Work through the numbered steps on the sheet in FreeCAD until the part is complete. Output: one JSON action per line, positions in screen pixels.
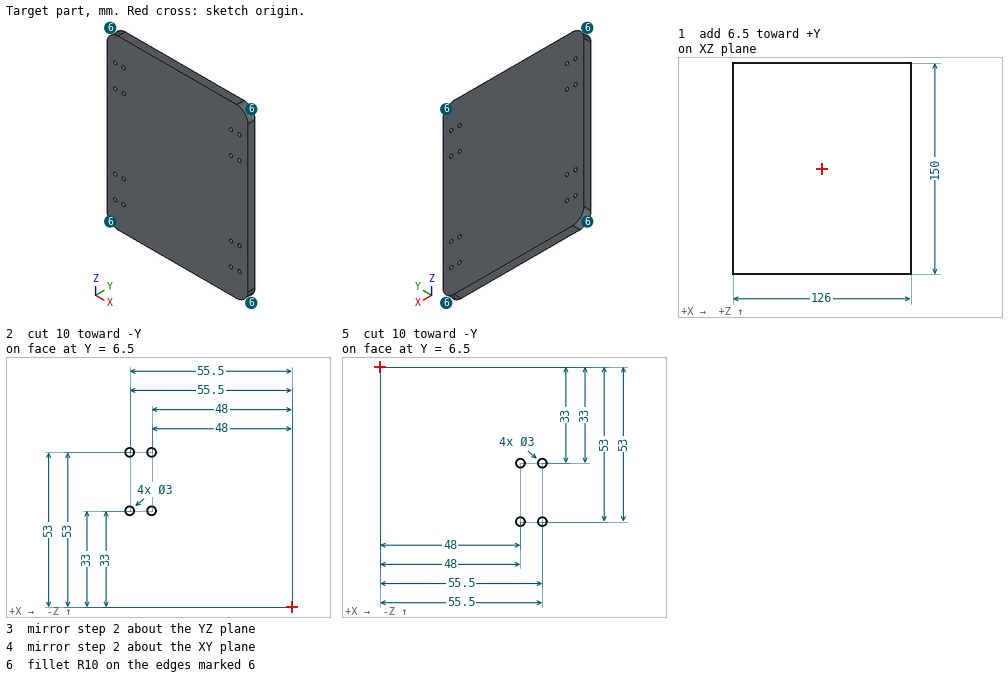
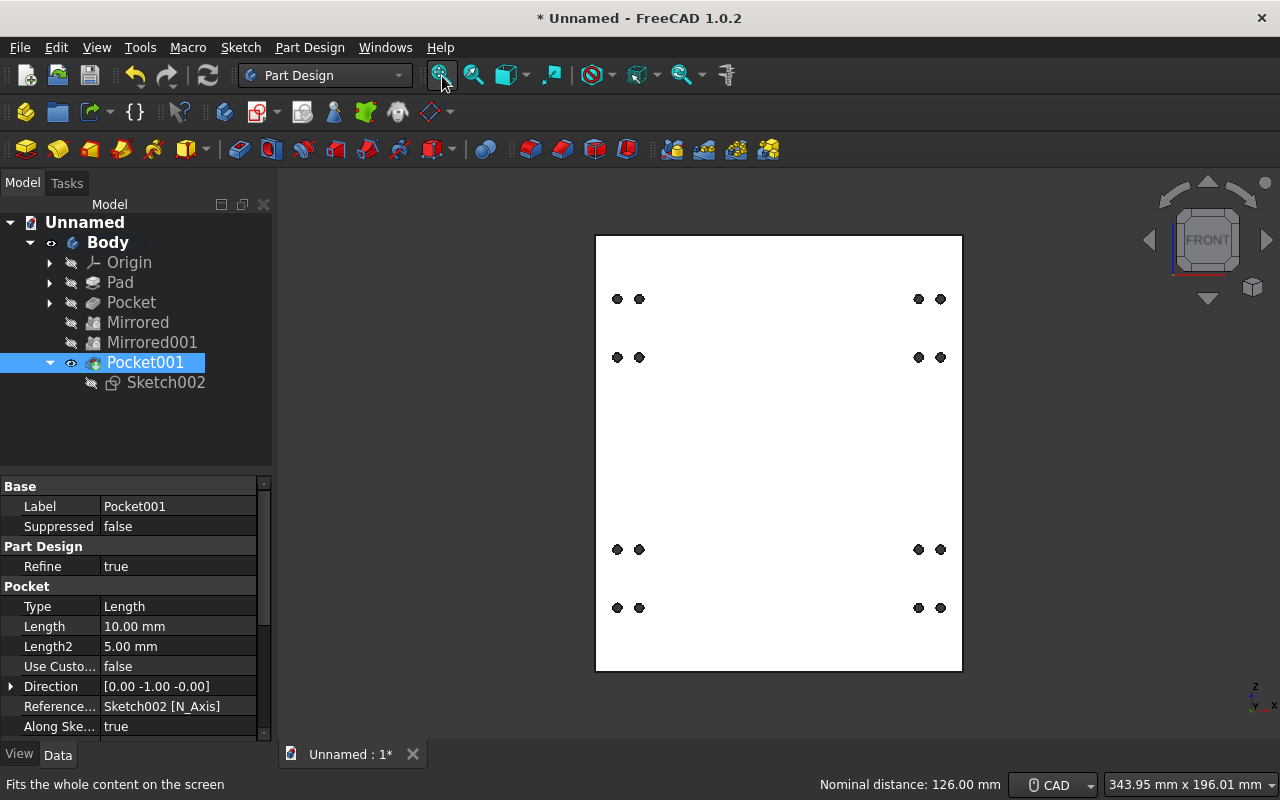
{"action": "scroll", "coordinate": [595, 671], "scroll_direction": "up", "scroll_amount": 4}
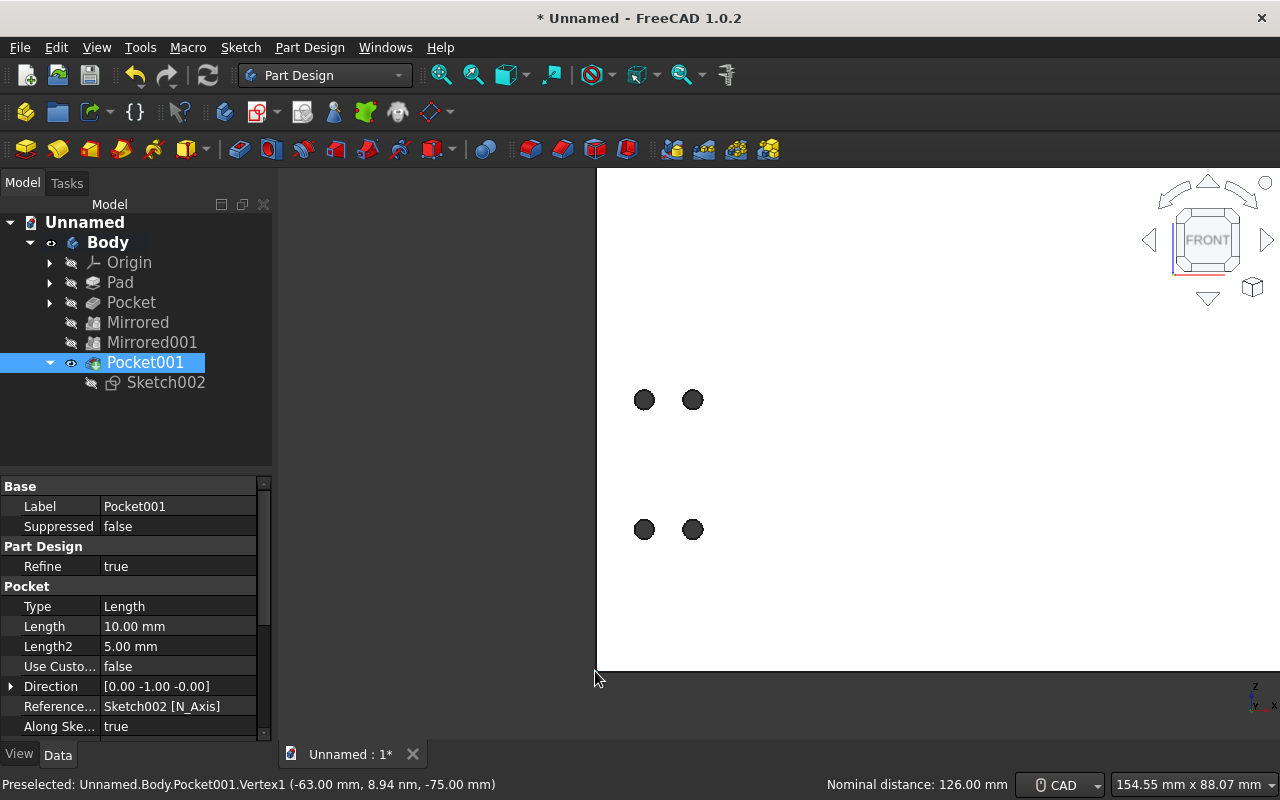
{"action": "key", "text": "v f"}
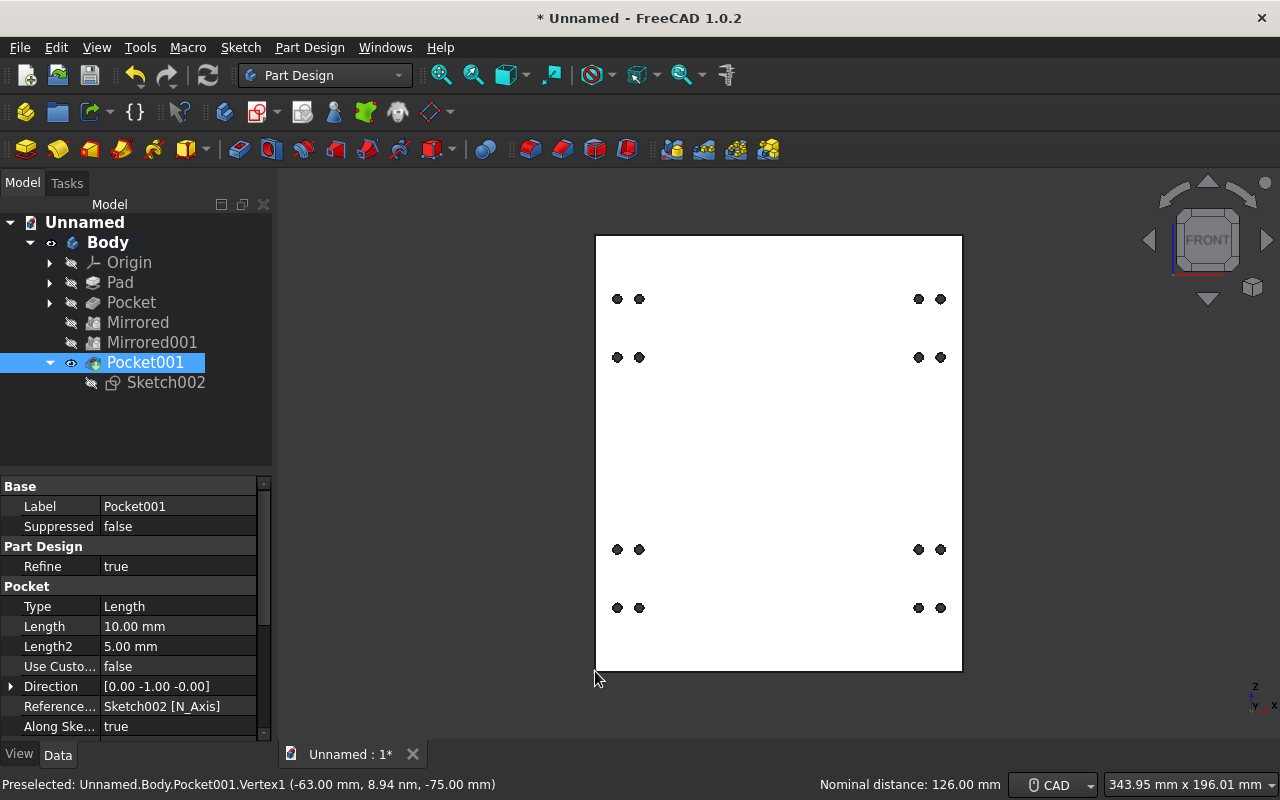
{"action": "key", "text": "3"}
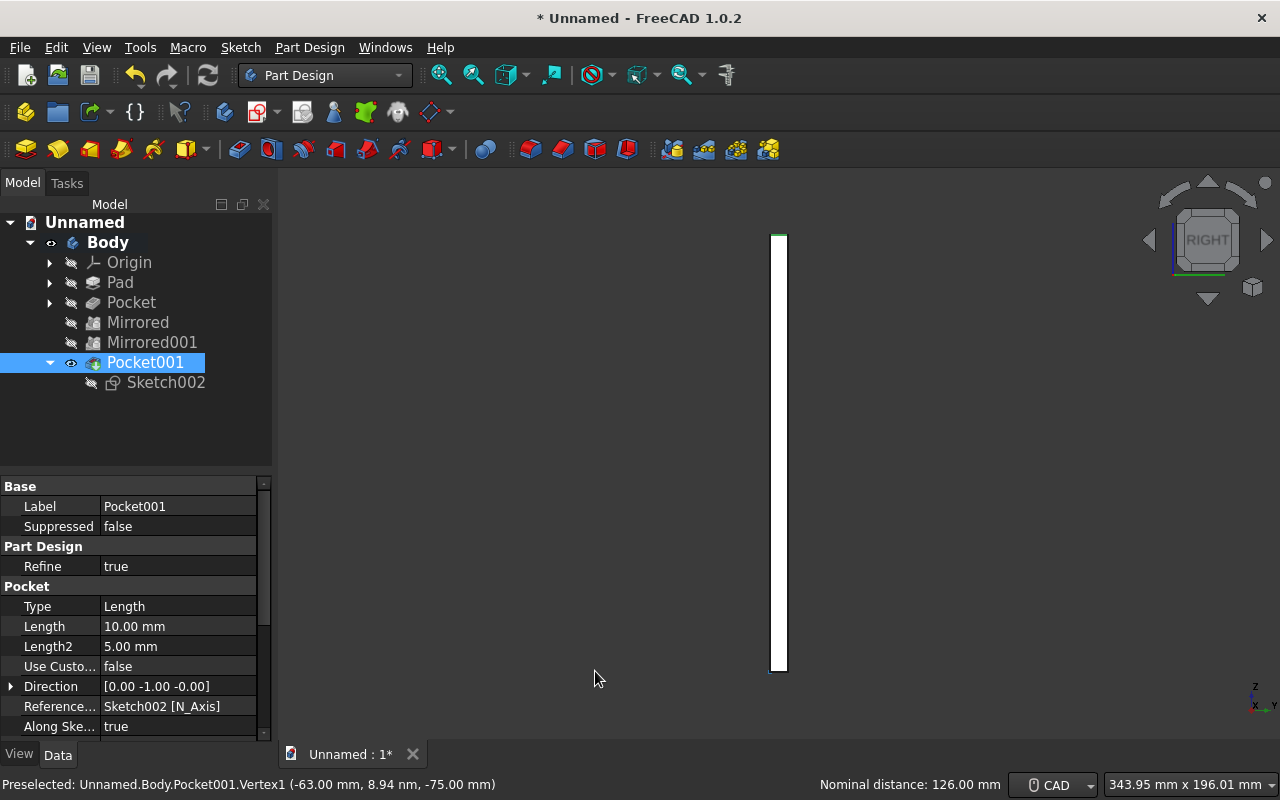
{"action": "left_click", "coordinate": [779, 671], "text": "ctrl"}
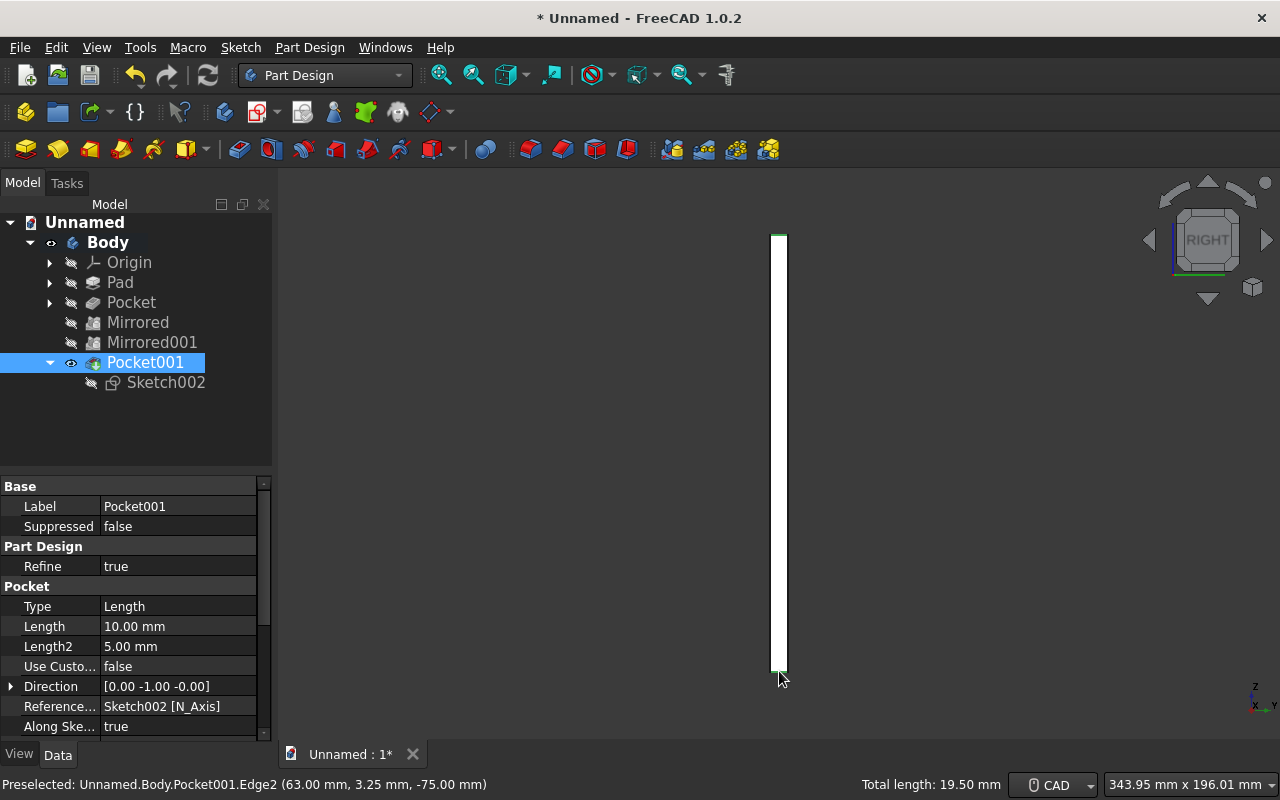
{"action": "scroll", "coordinate": [779, 671], "scroll_direction": "up", "scroll_amount": 4}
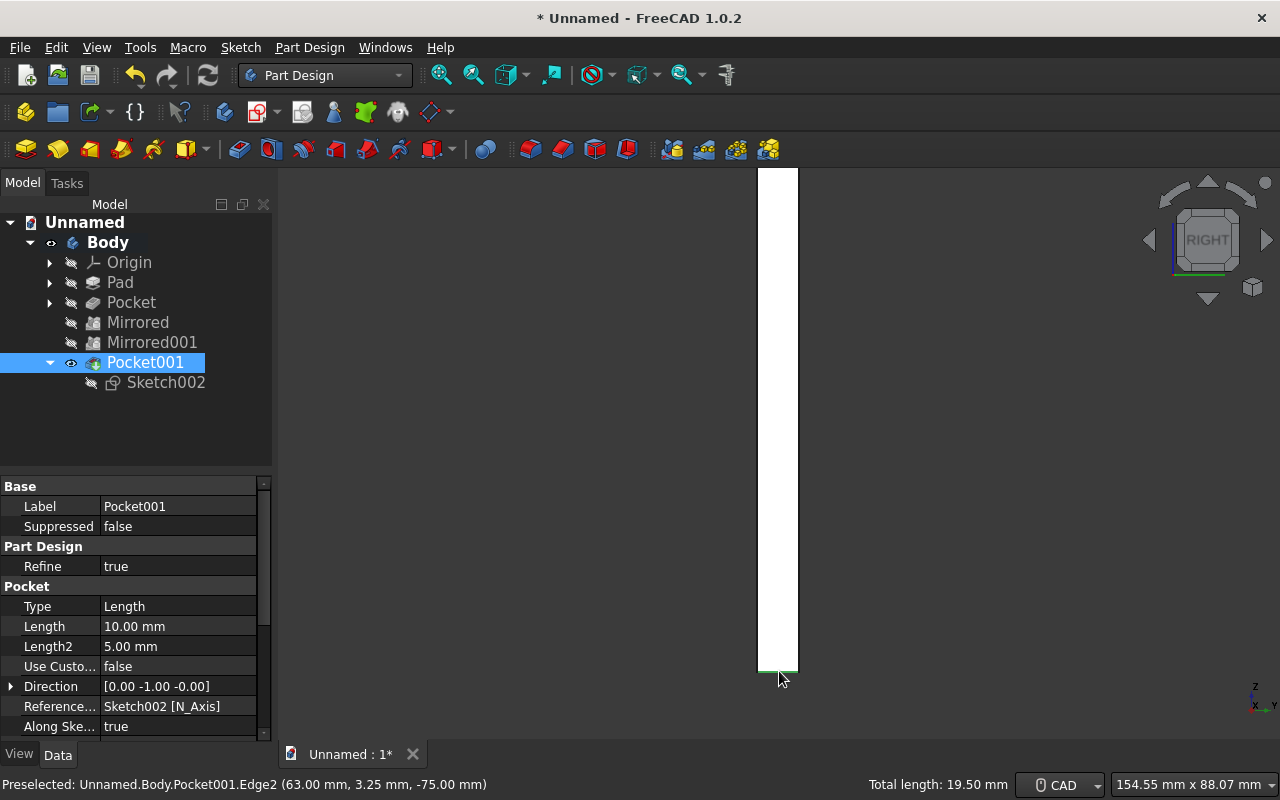
{"action": "left_click", "coordinate": [442, 76]}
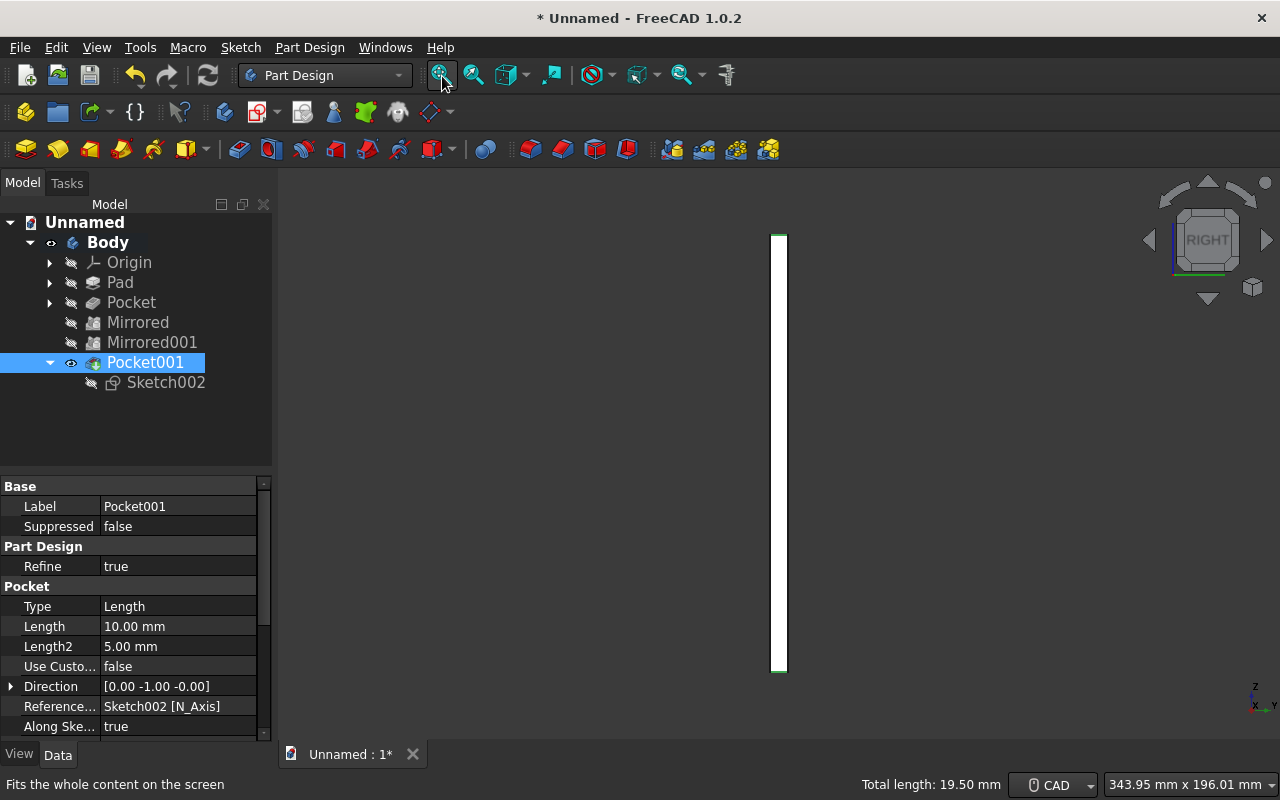
{"action": "key", "text": "5"}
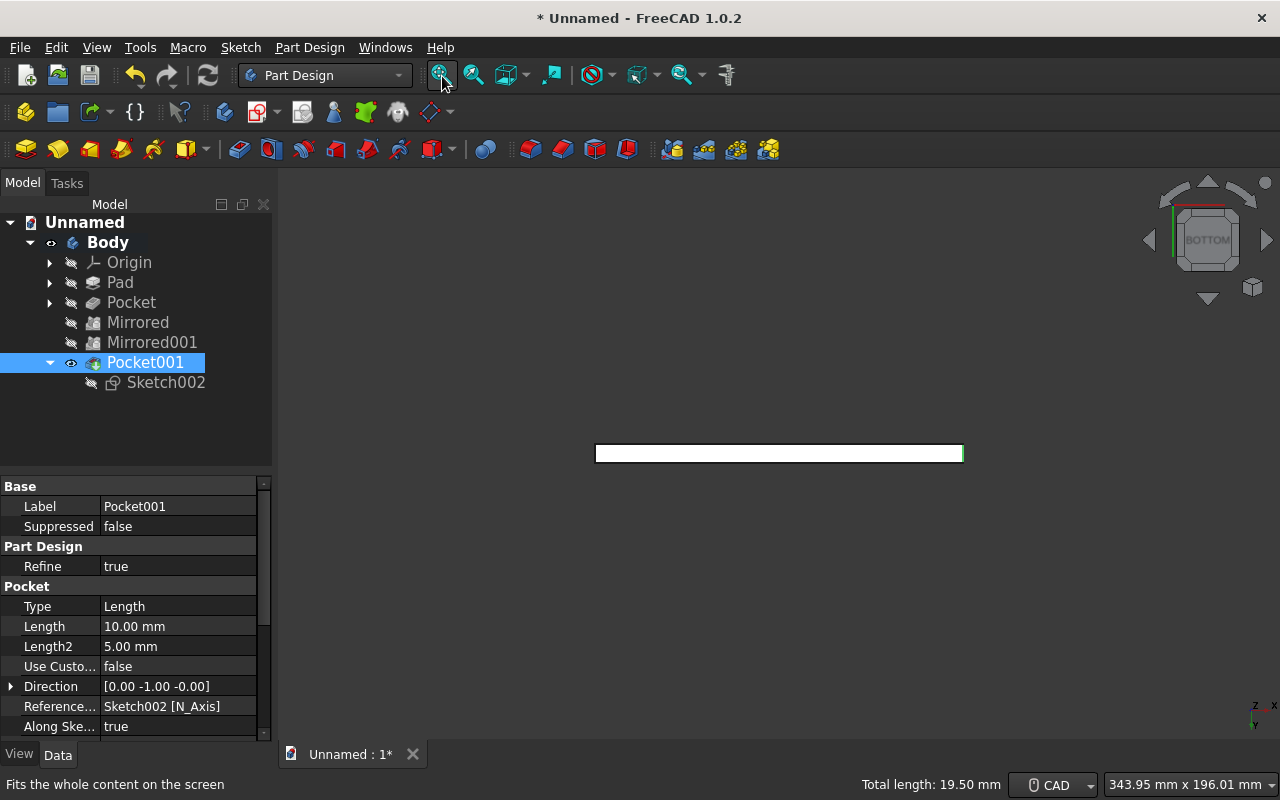
{"action": "left_click", "coordinate": [442, 76]}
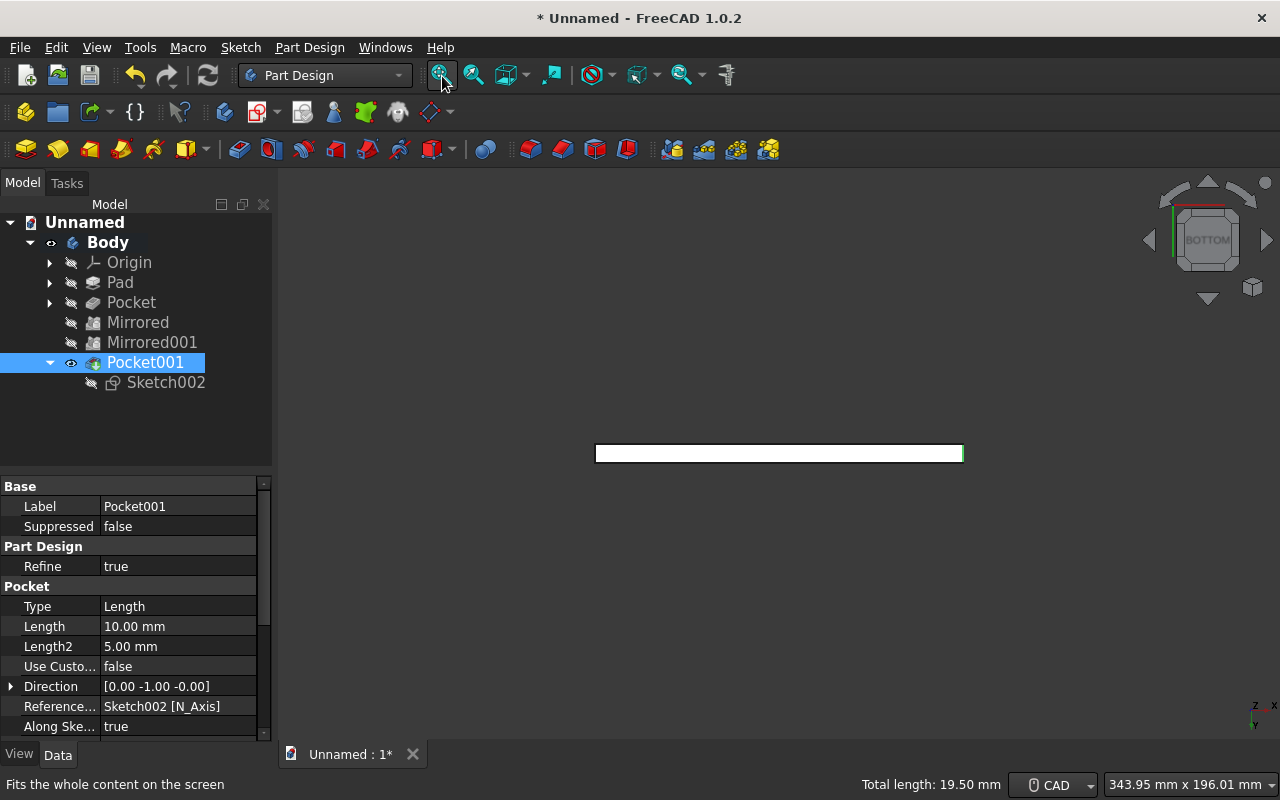
{"action": "left_click", "coordinate": [595, 452], "text": "ctrl"}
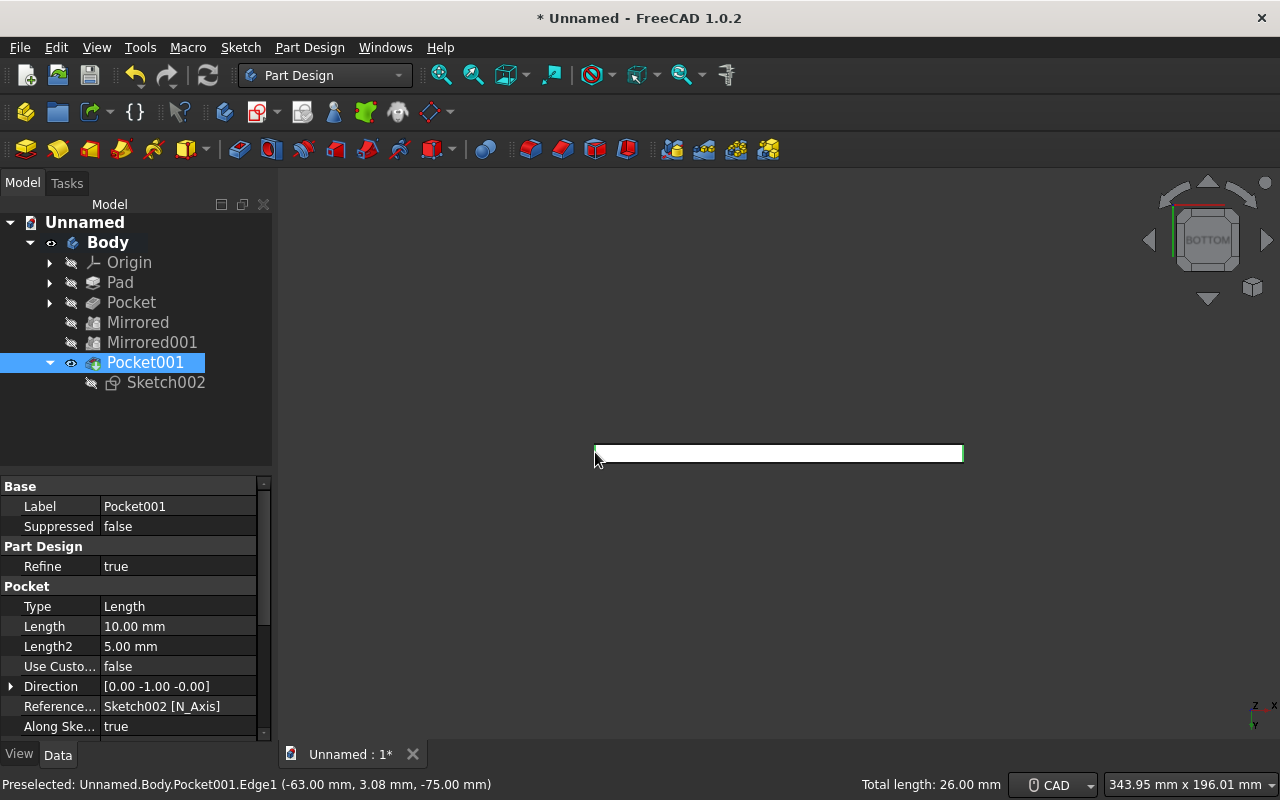
{"action": "left_click", "coordinate": [532, 150]}